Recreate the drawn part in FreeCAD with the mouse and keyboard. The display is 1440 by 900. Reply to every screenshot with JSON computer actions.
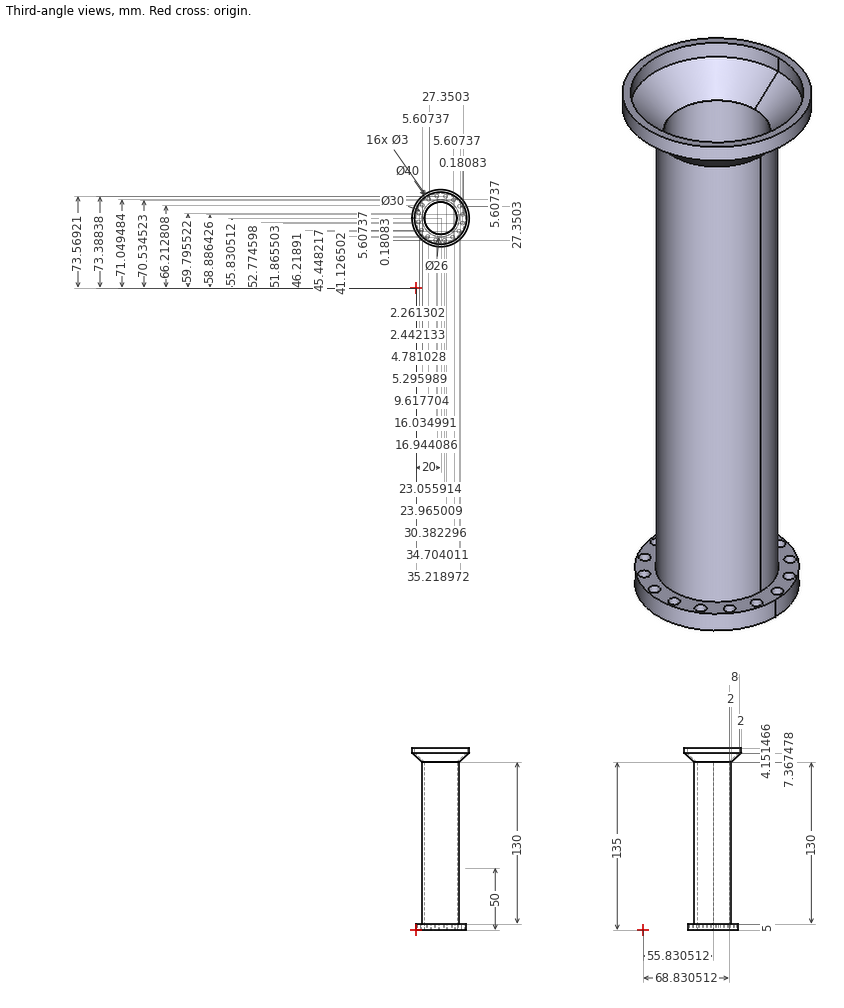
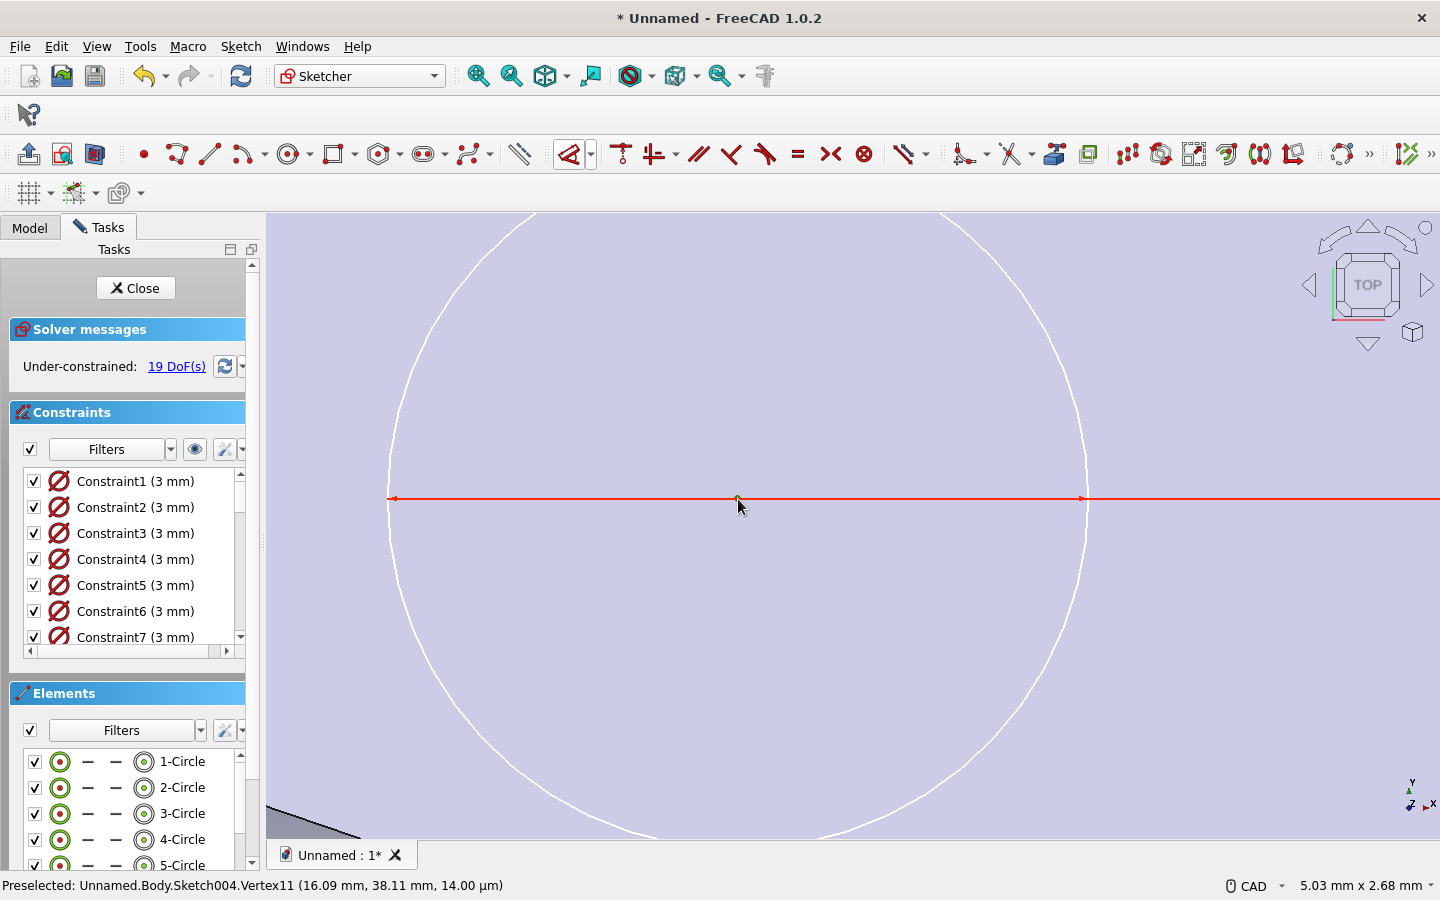
{"action": "left_click", "coordinate": [590, 154]}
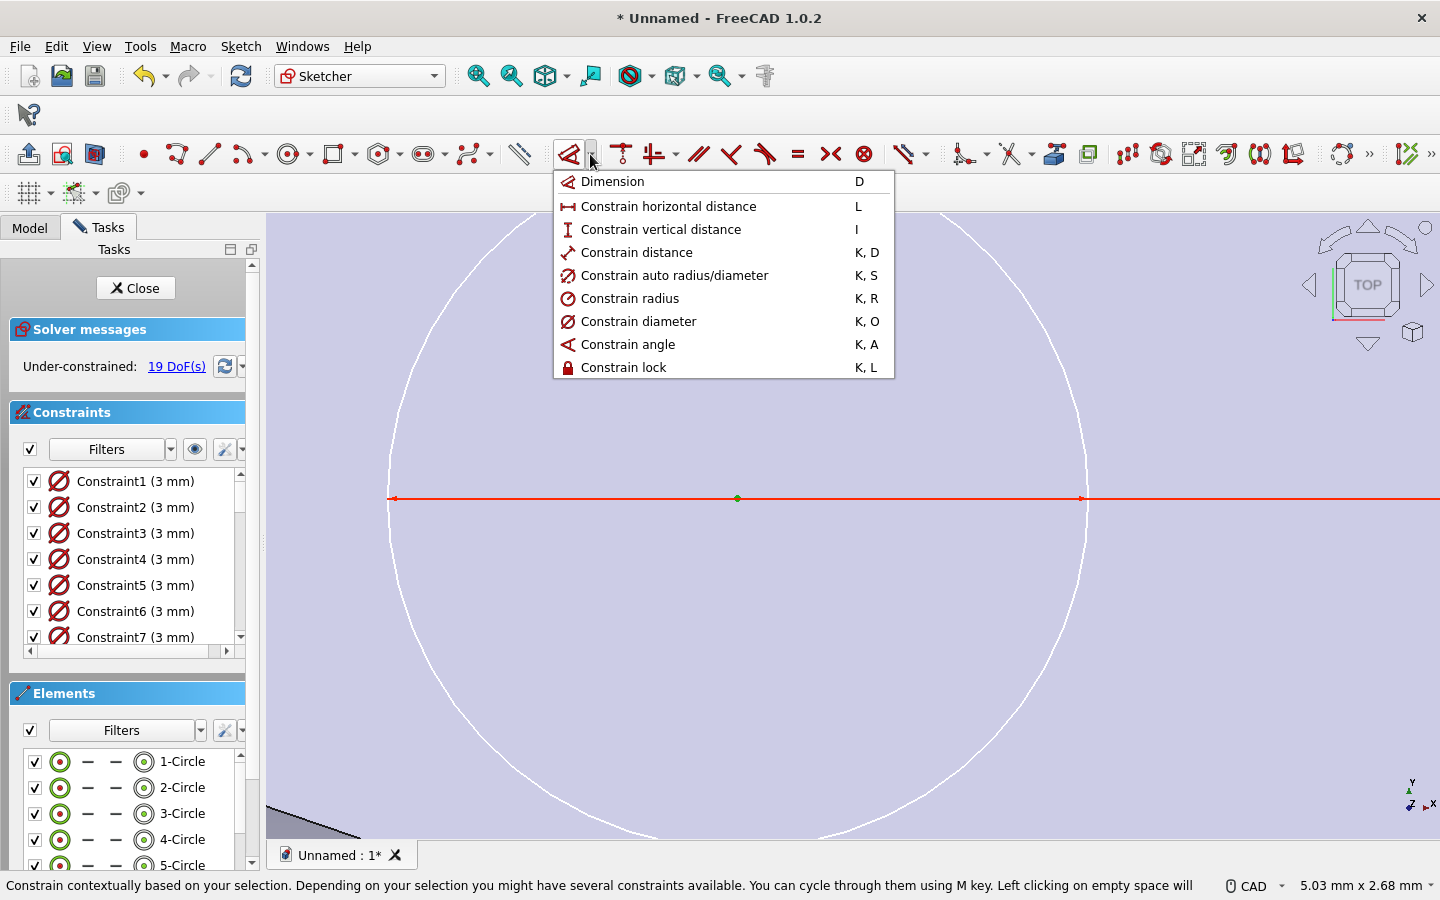
{"action": "left_click", "coordinate": [724, 230]}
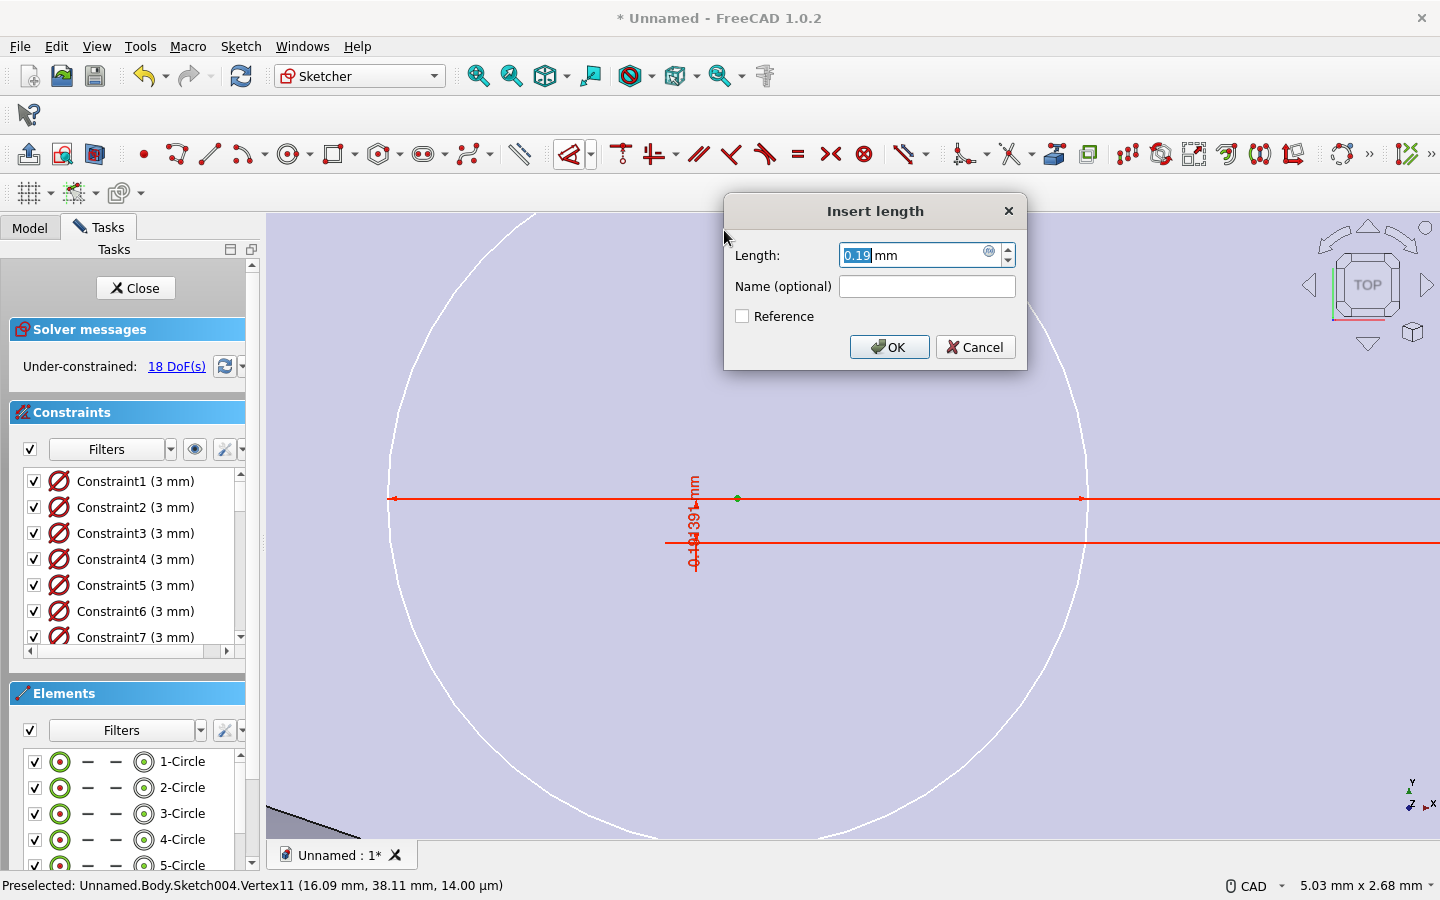
{"action": "type", "text": "0.18083"}
{"action": "key", "text": "Return"}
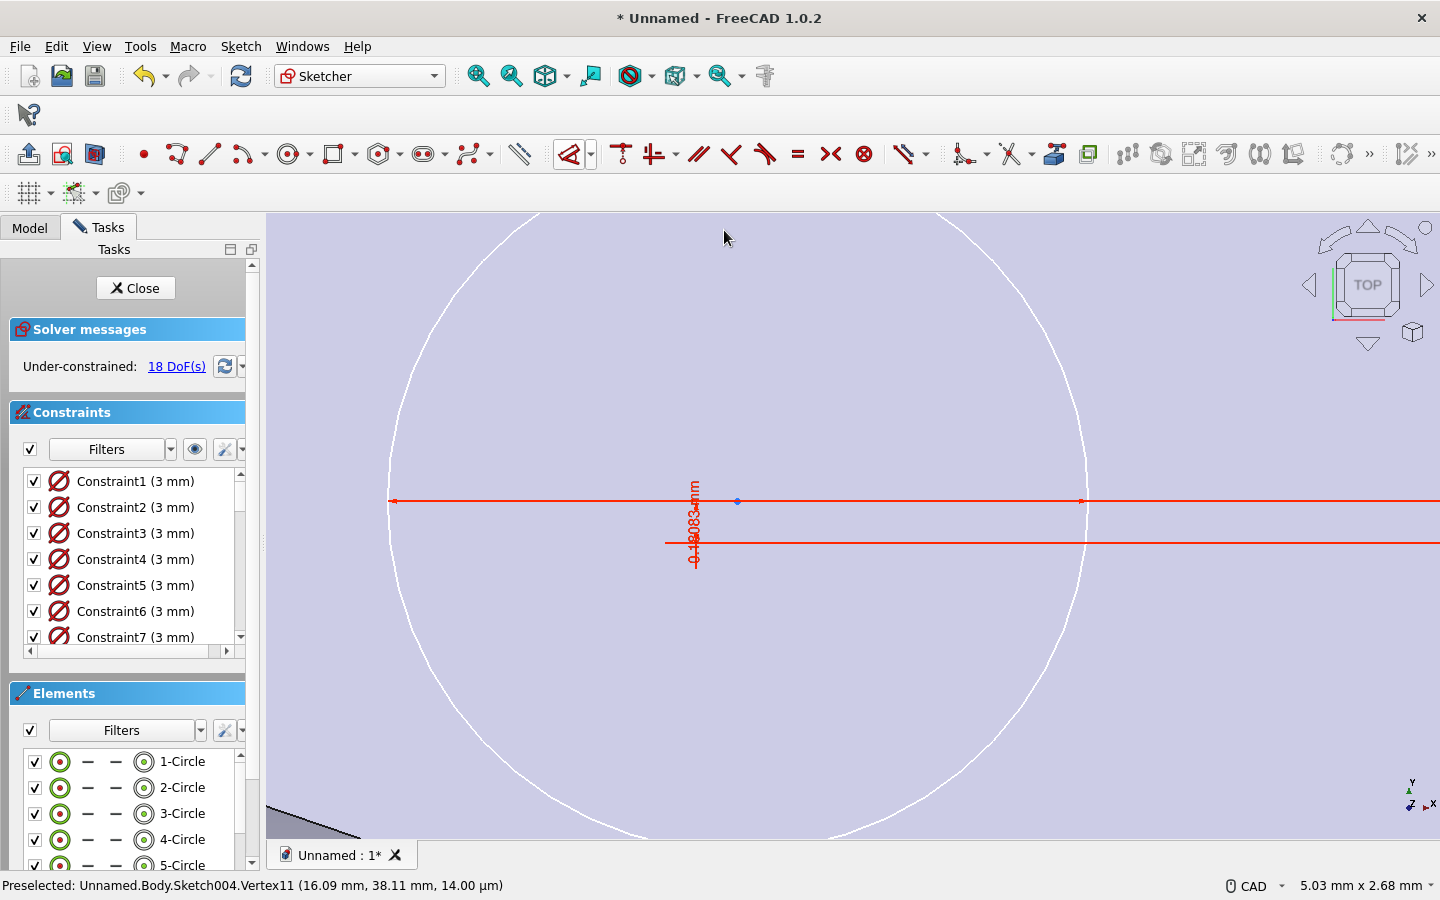
{"action": "scroll", "coordinate": [763, 523], "scroll_direction": "down", "scroll_amount": 18}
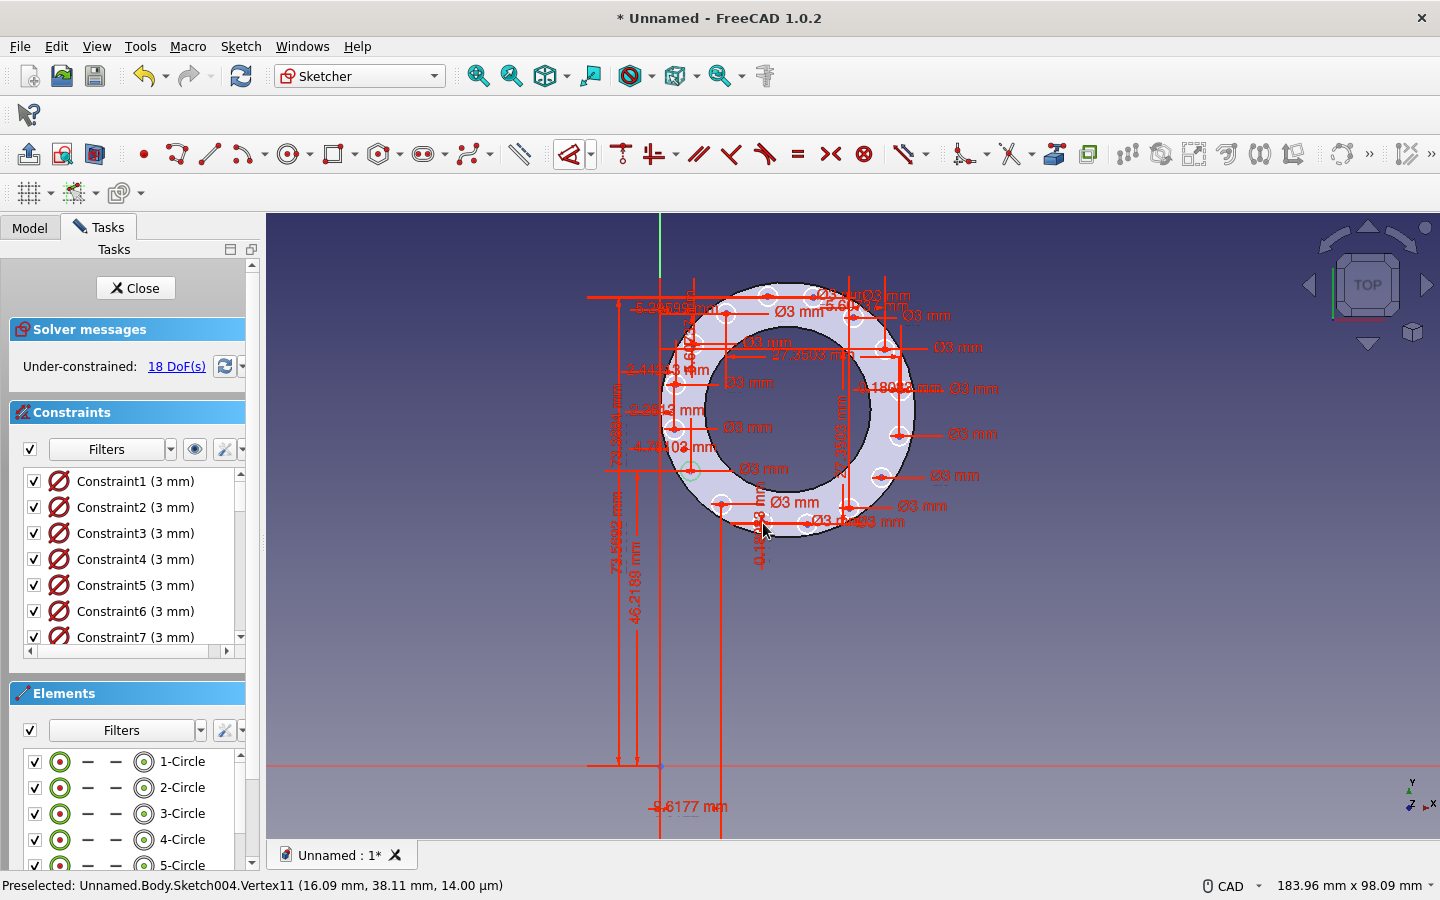
{"action": "left_click", "coordinate": [726, 314]}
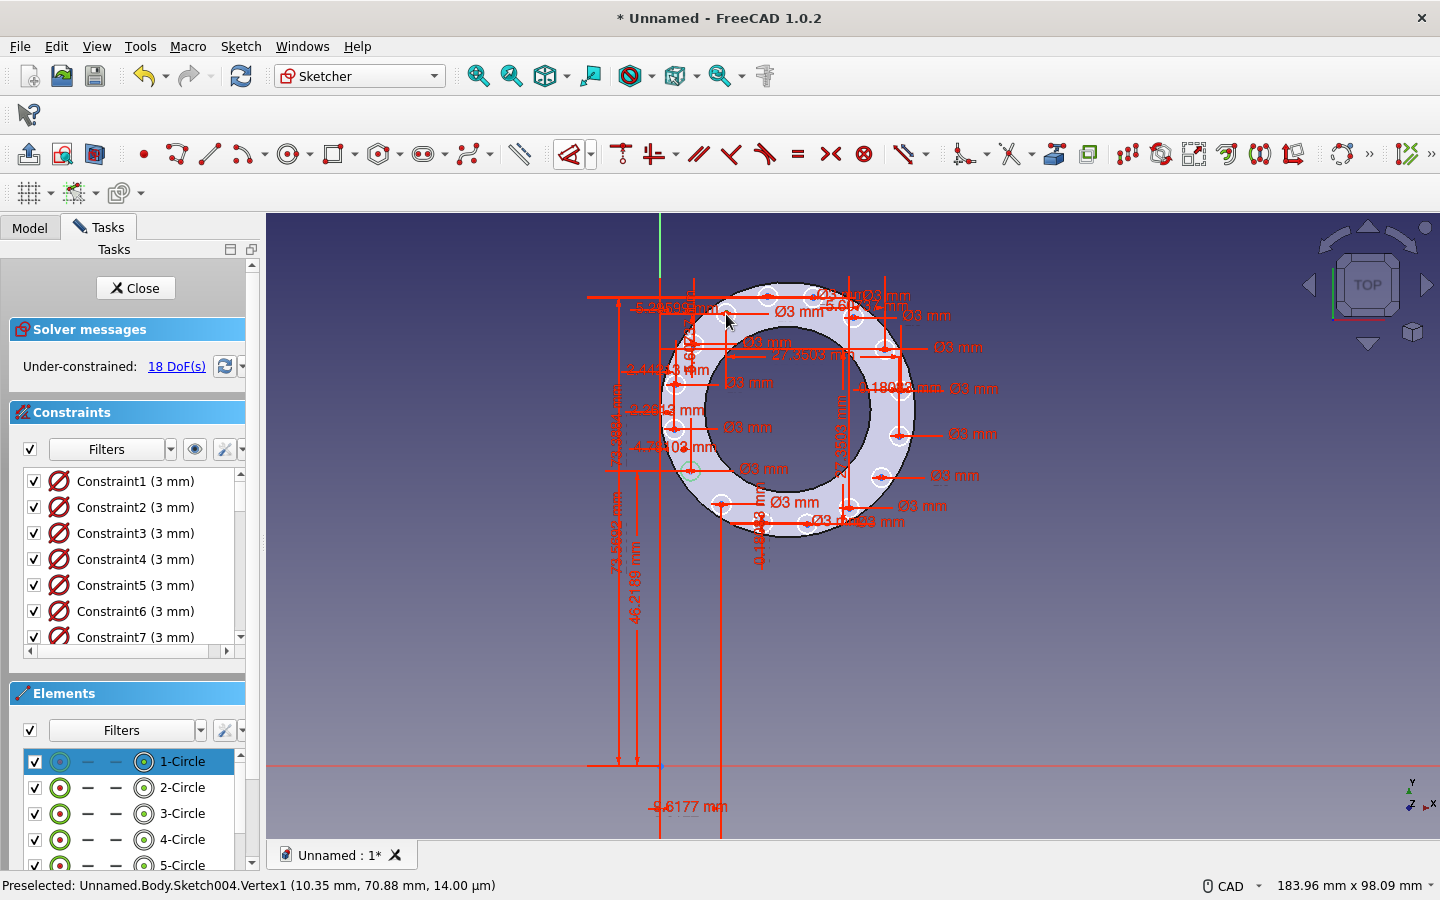
{"action": "left_click", "coordinate": [691, 471]}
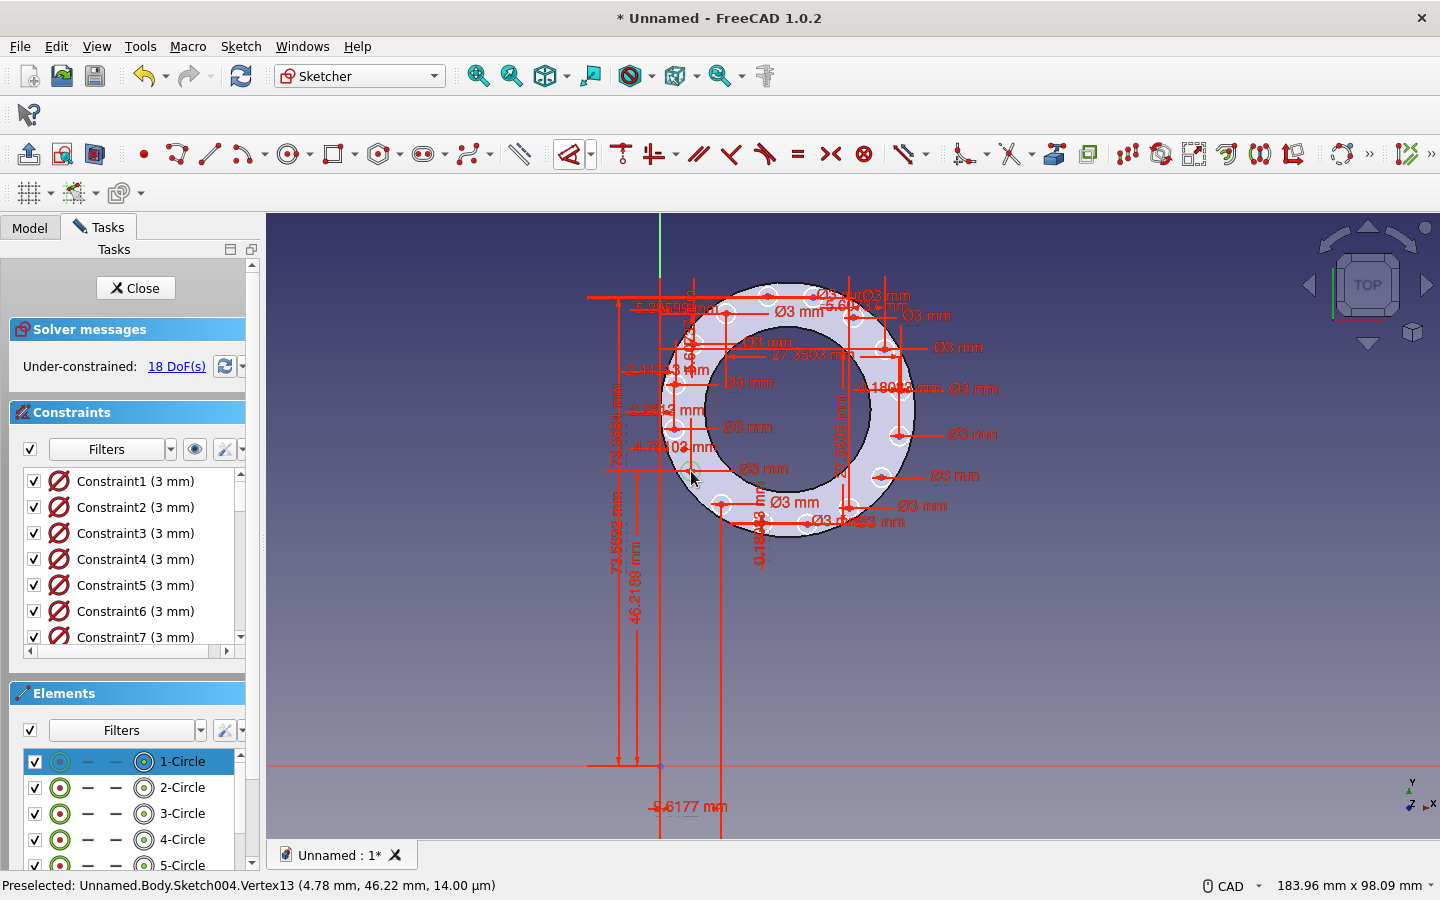
{"action": "key", "text": "l"}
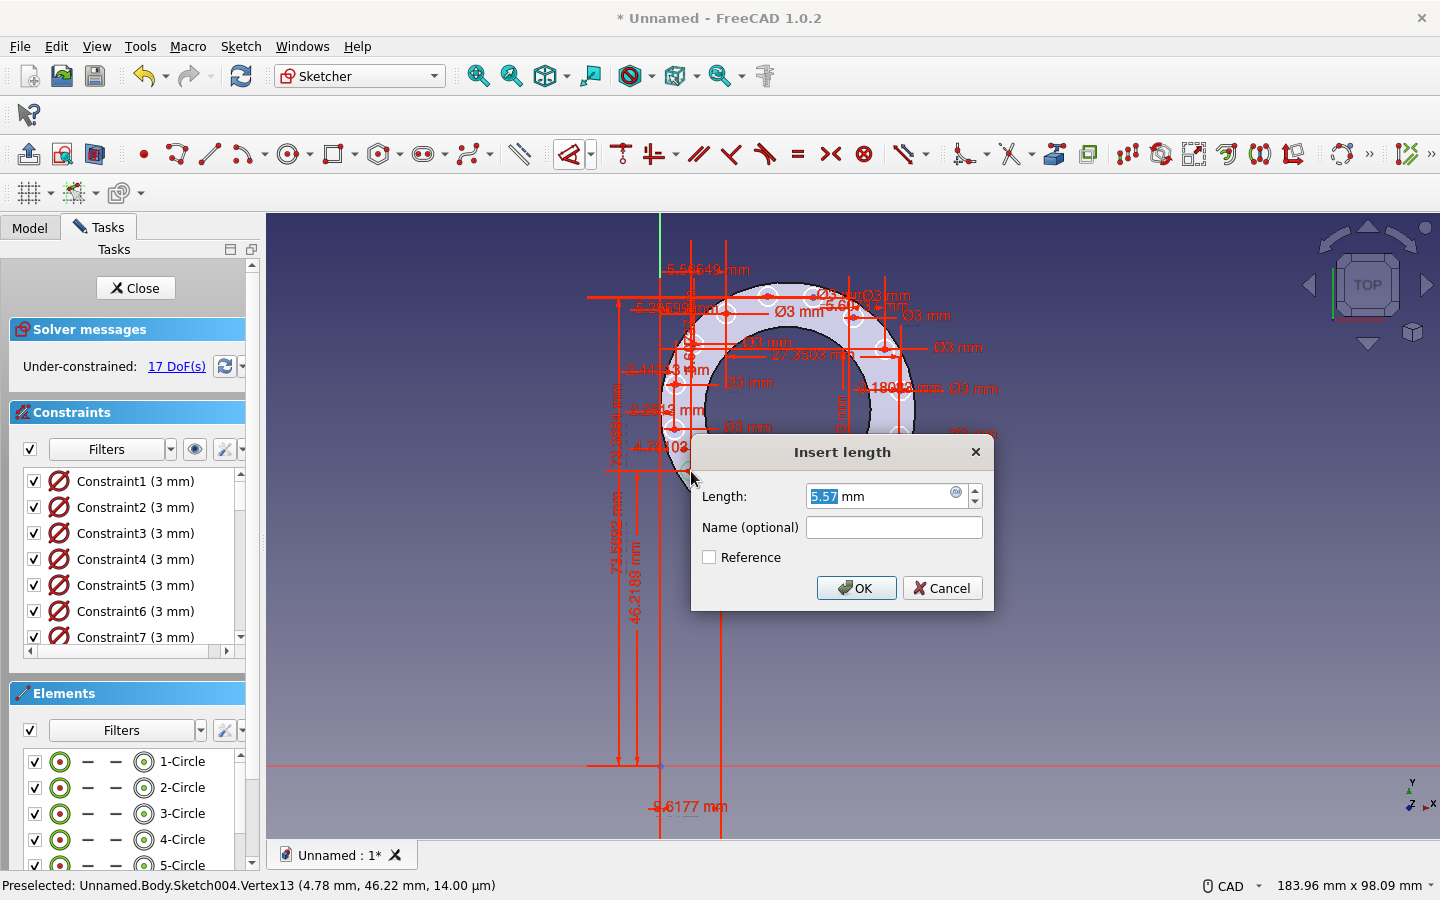
{"action": "type", "text": "5.60737"}
{"action": "key", "text": "Return"}